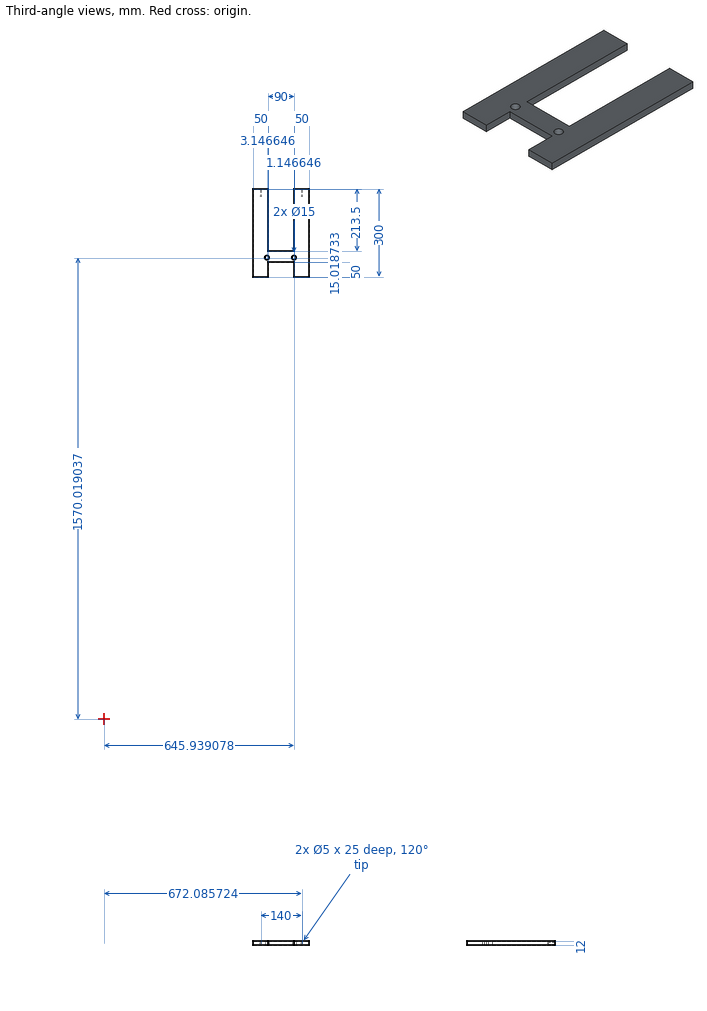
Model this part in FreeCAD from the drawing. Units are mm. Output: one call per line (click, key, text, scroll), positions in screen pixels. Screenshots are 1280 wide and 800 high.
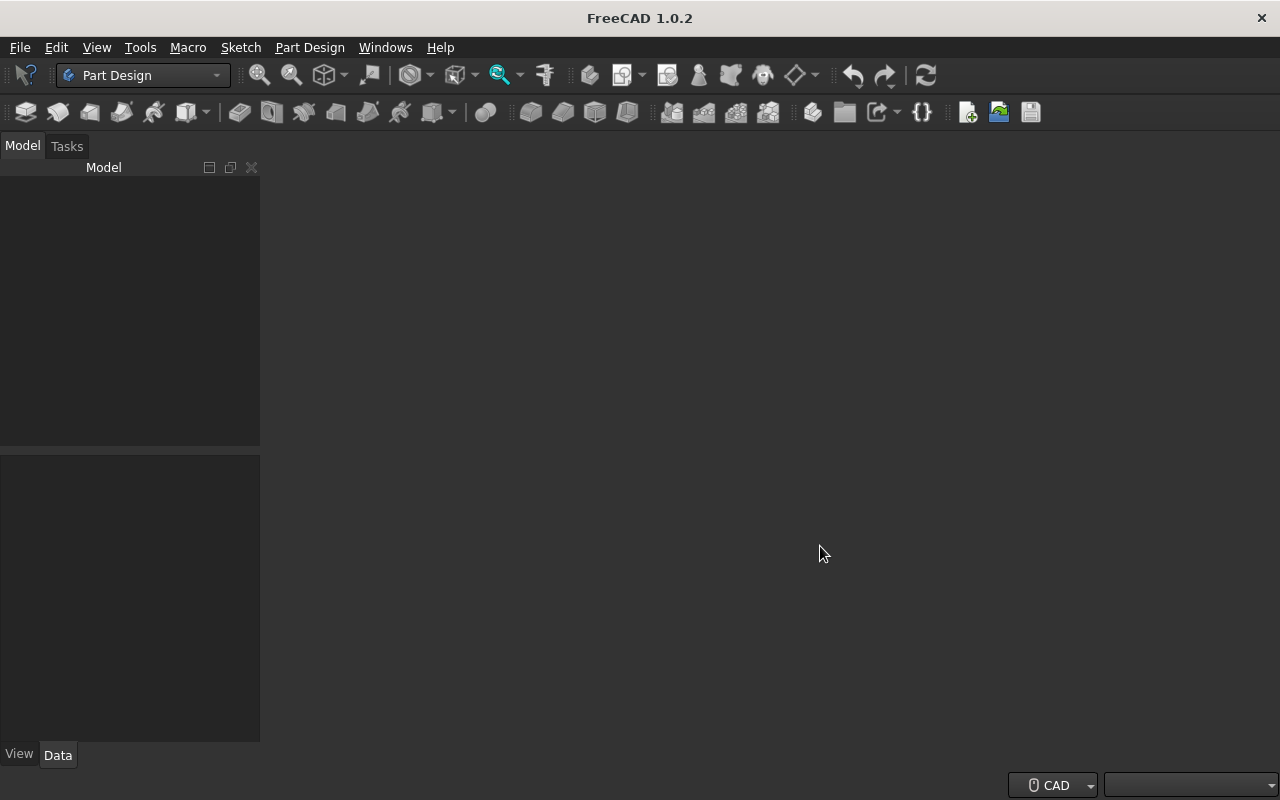
key(ctrl+n)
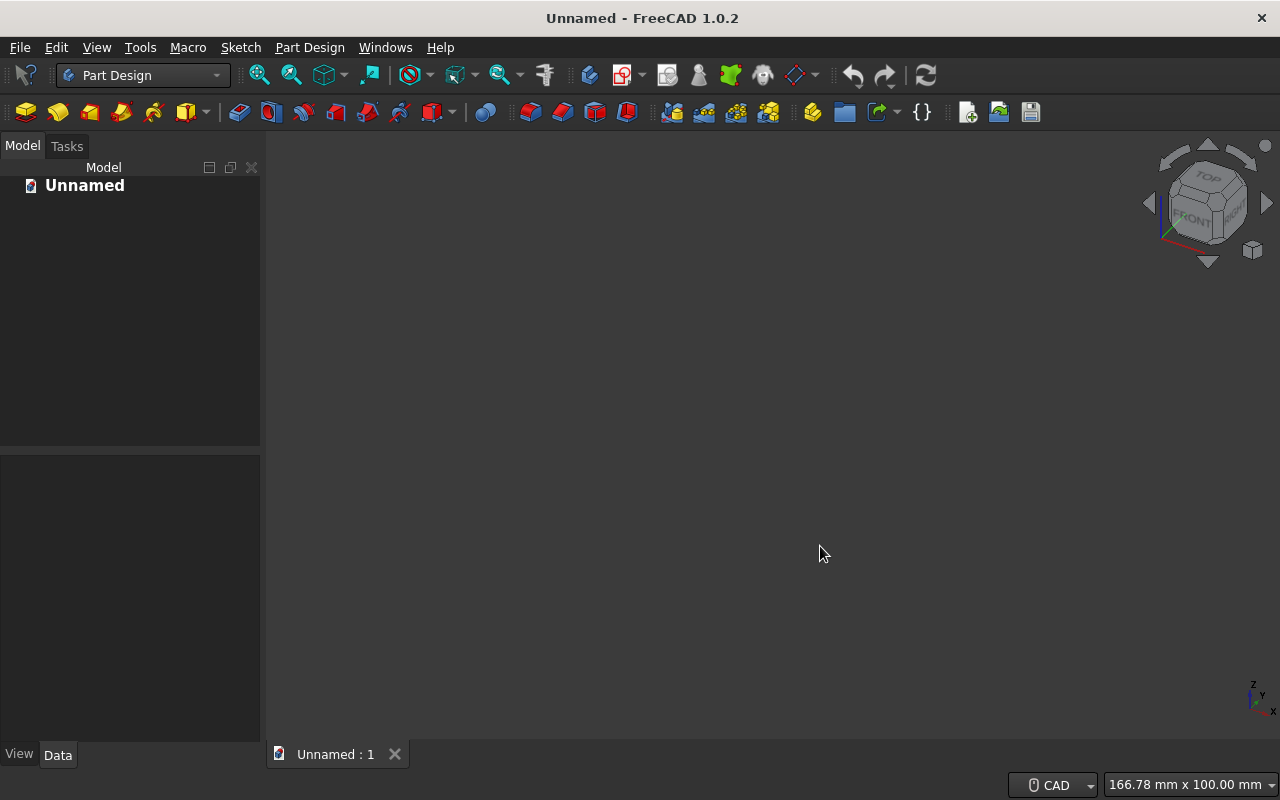
click(590, 76)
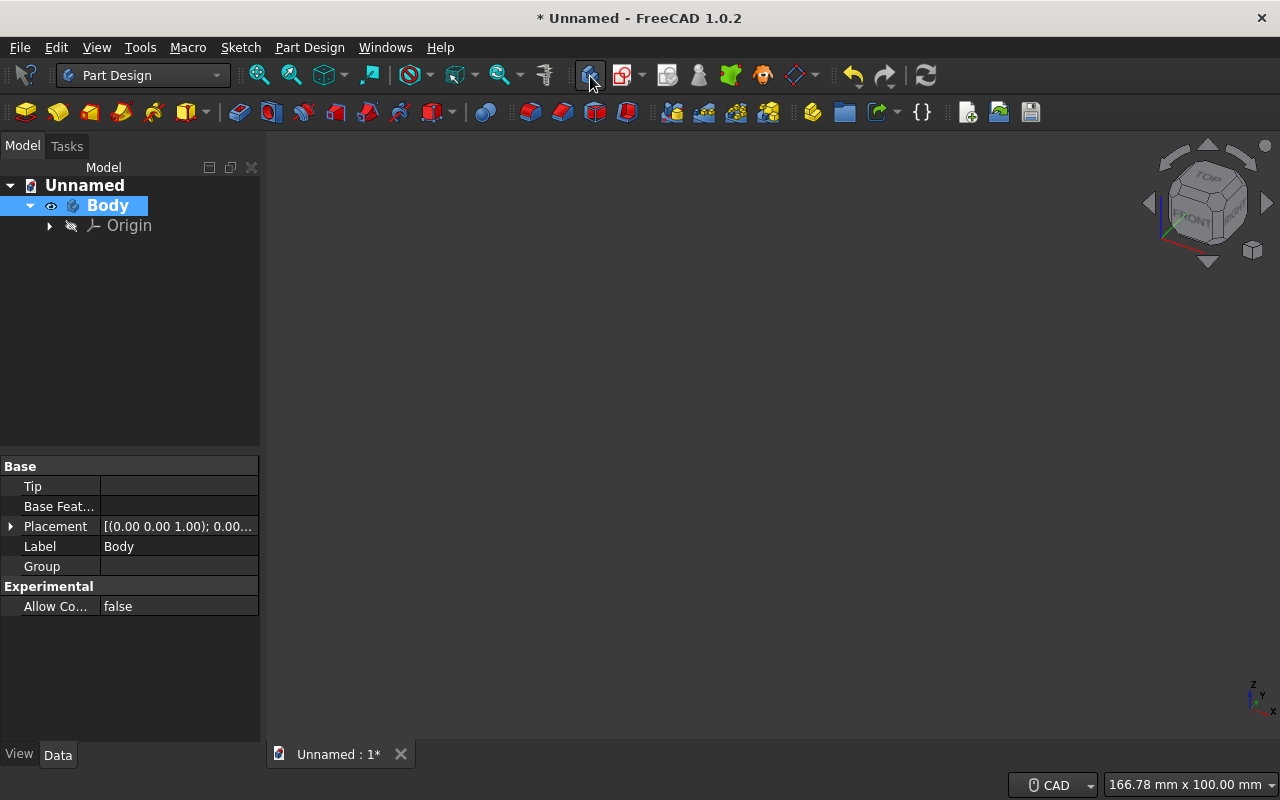
click(50, 226)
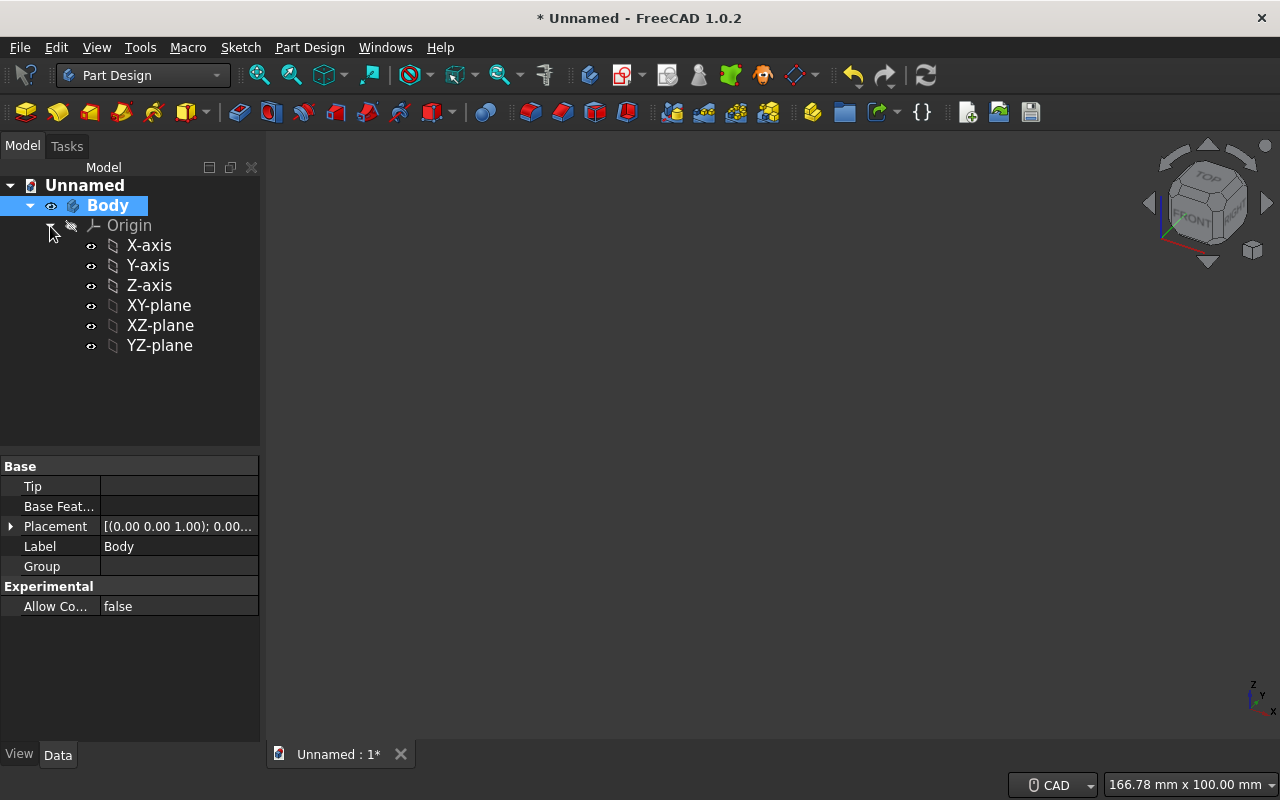
click(136, 306)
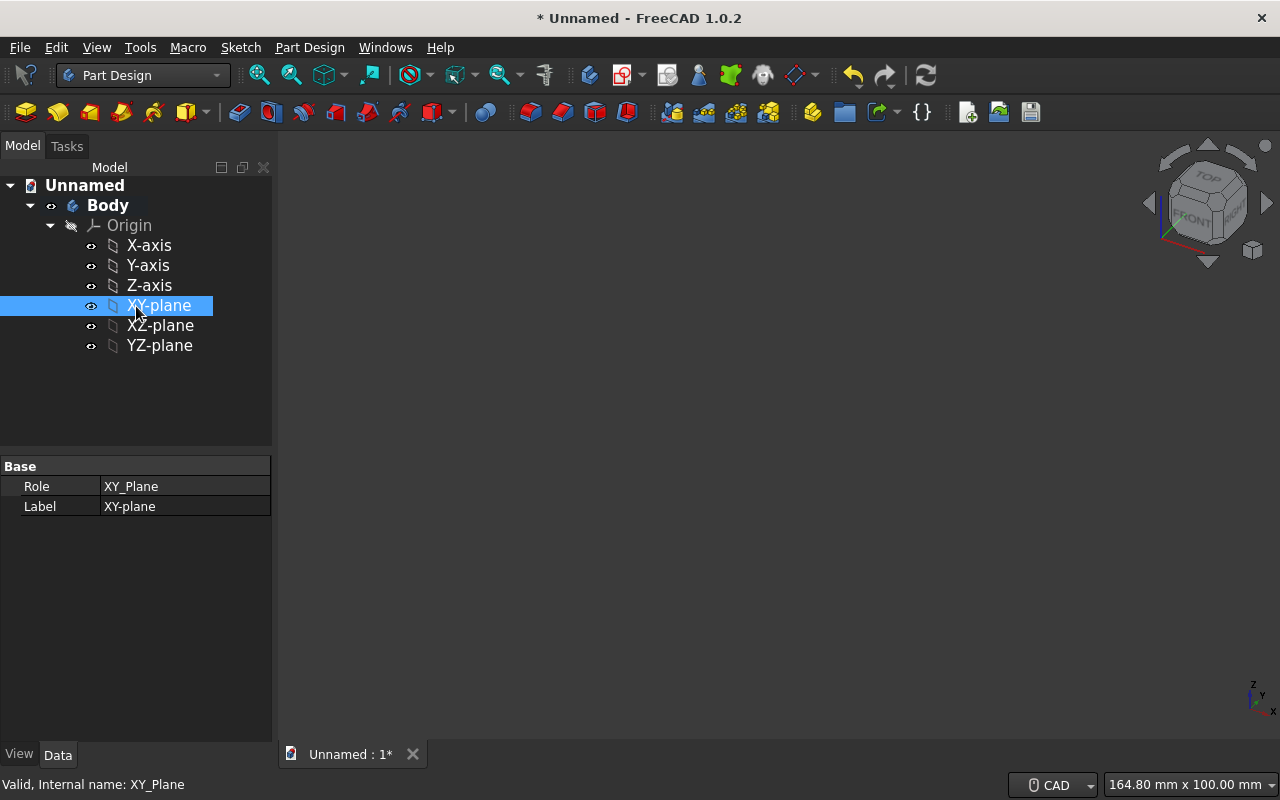
click(796, 76)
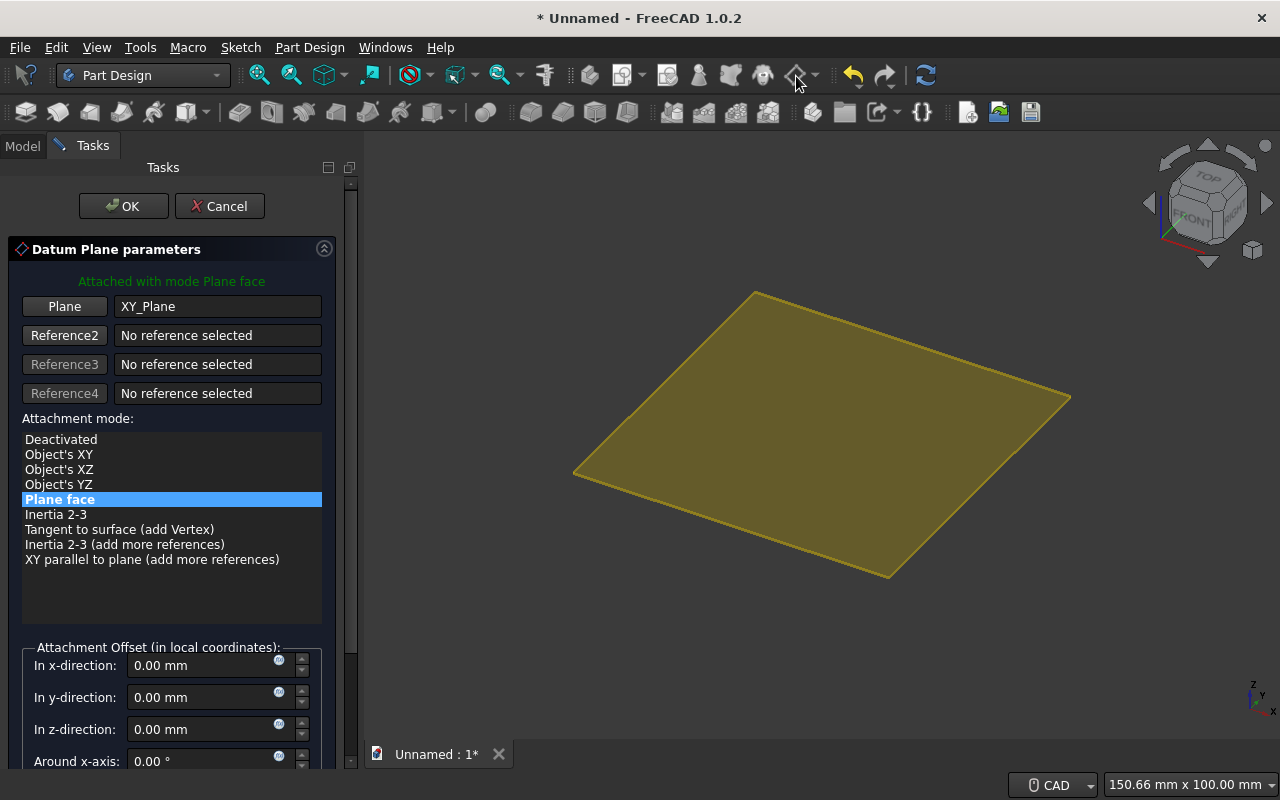
triple_click(210, 729)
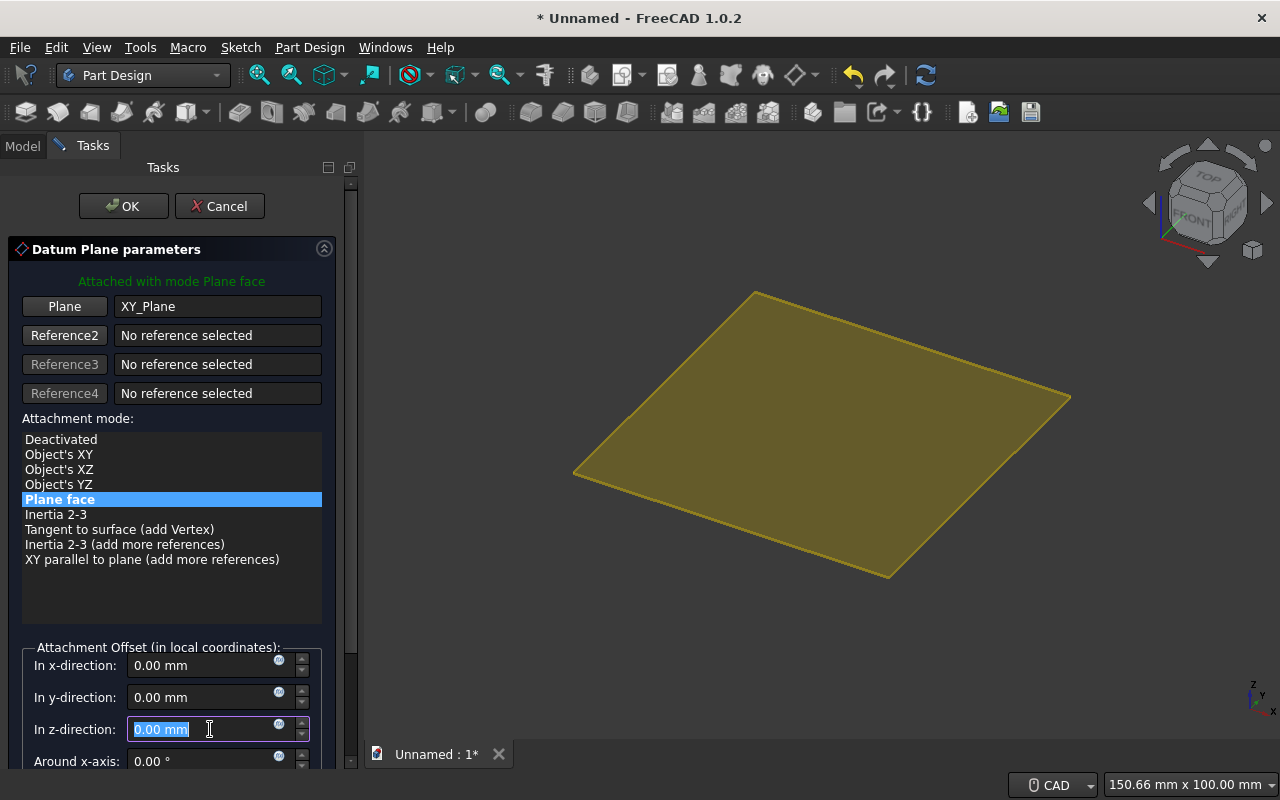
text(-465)
key(Tab)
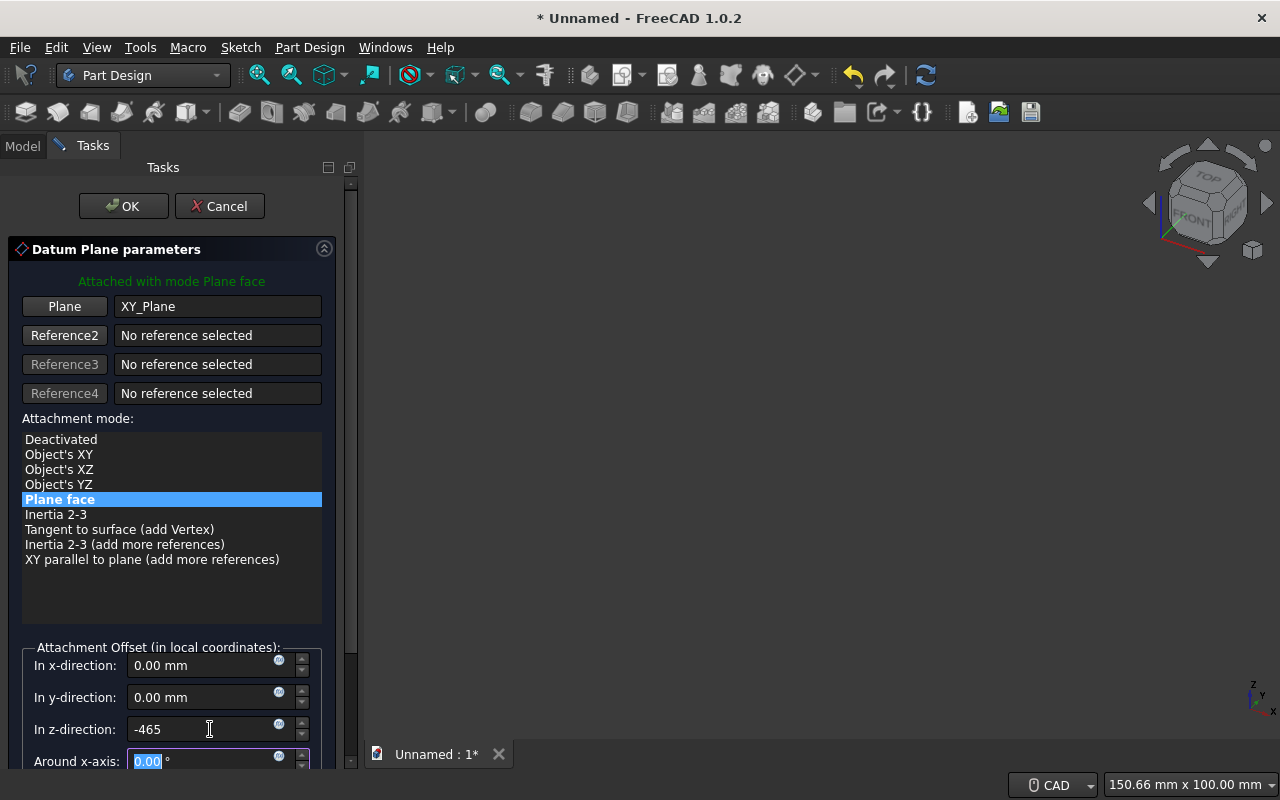
click(124, 206)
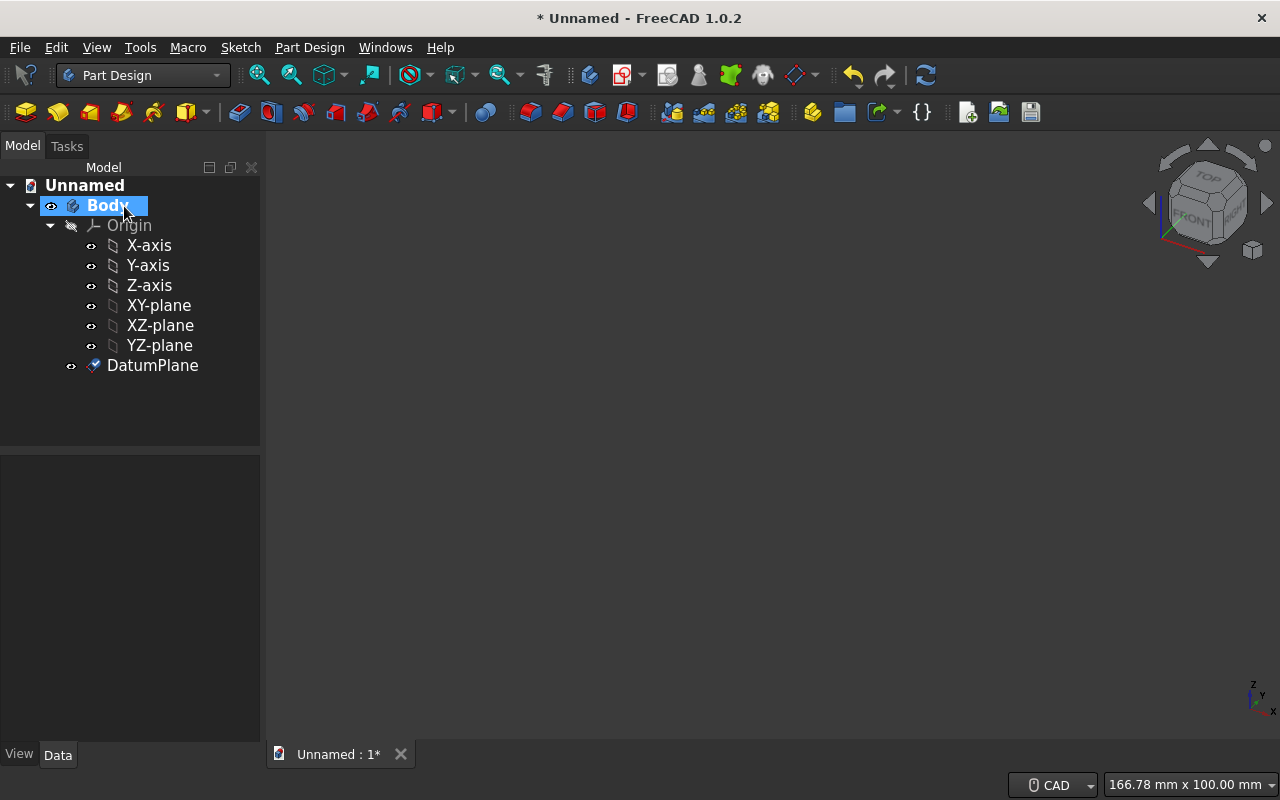
click(116, 366)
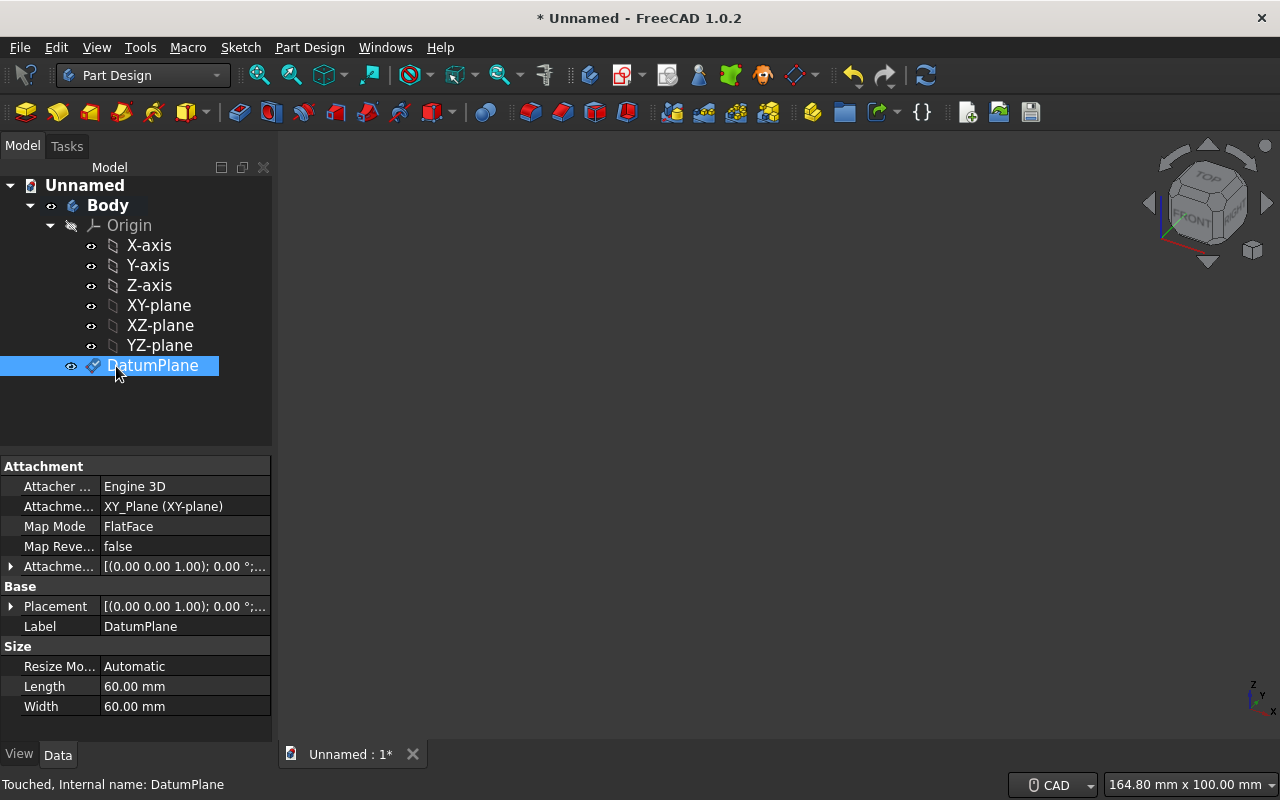
click(622, 76)